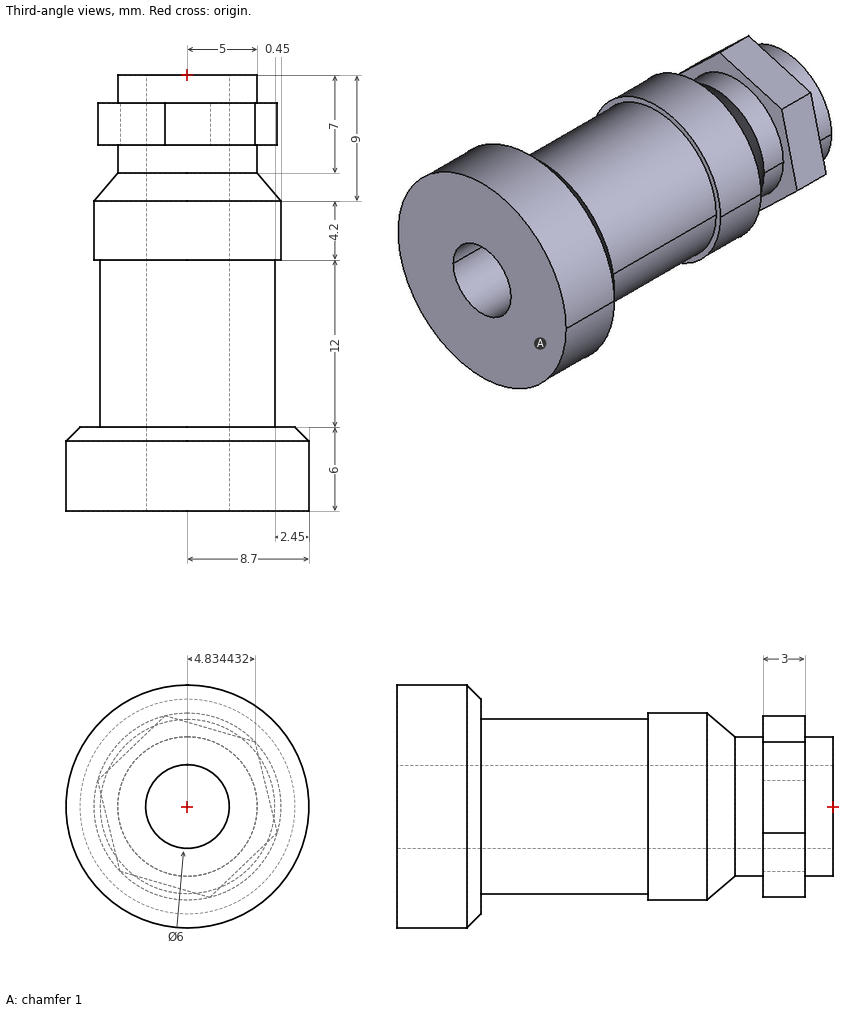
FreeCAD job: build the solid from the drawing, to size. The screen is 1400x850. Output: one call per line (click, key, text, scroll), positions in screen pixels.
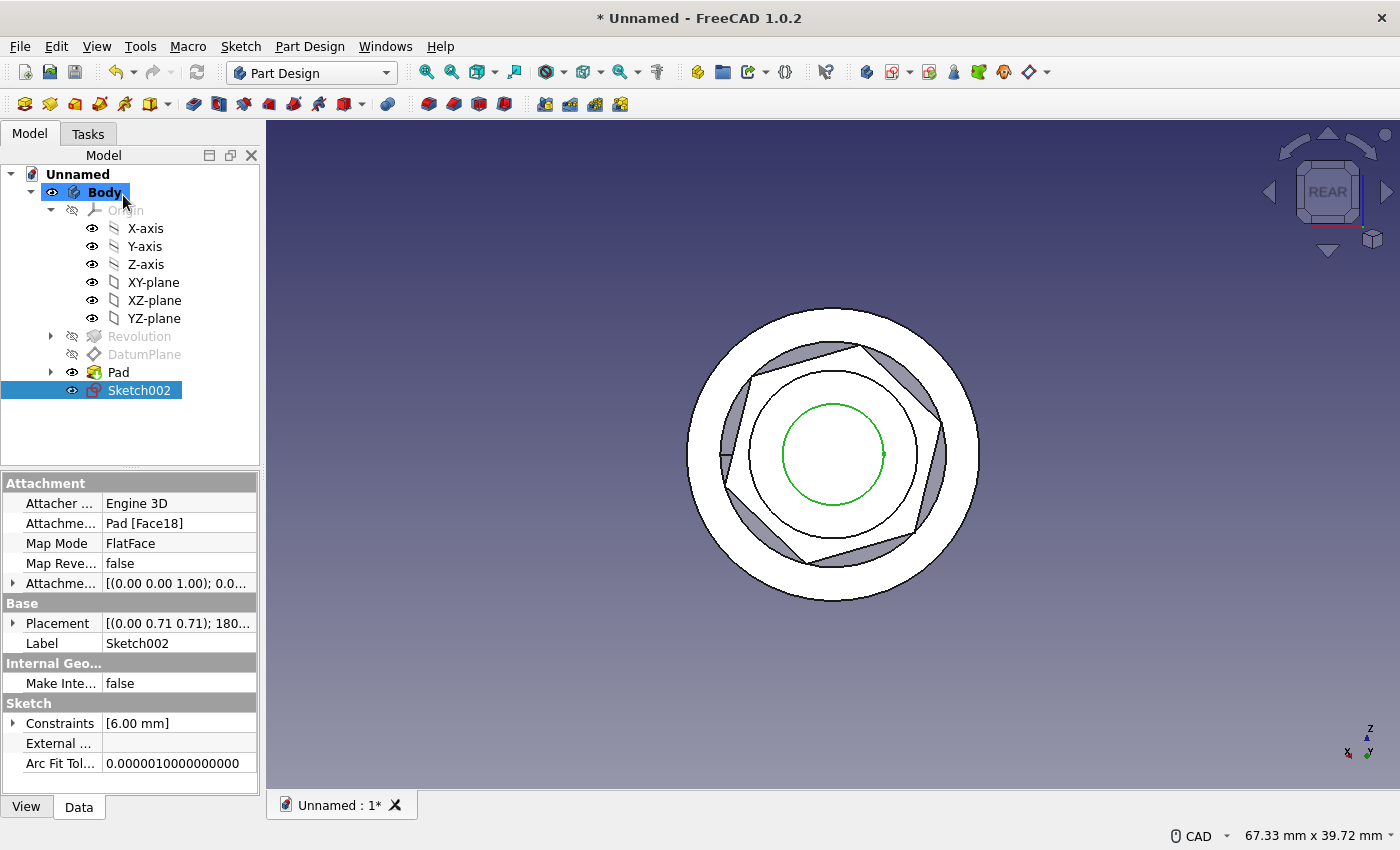
click(194, 104)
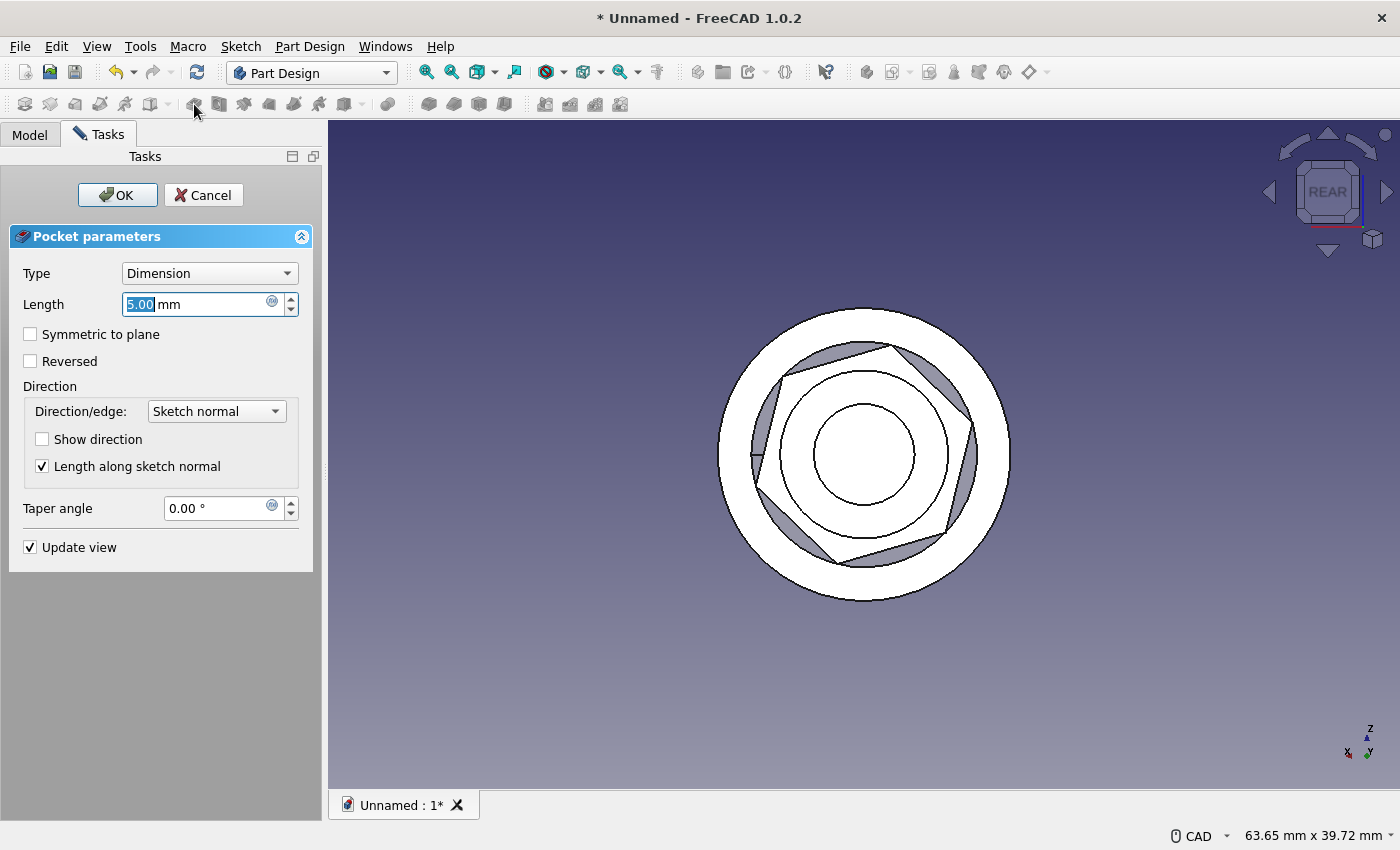
click(210, 274)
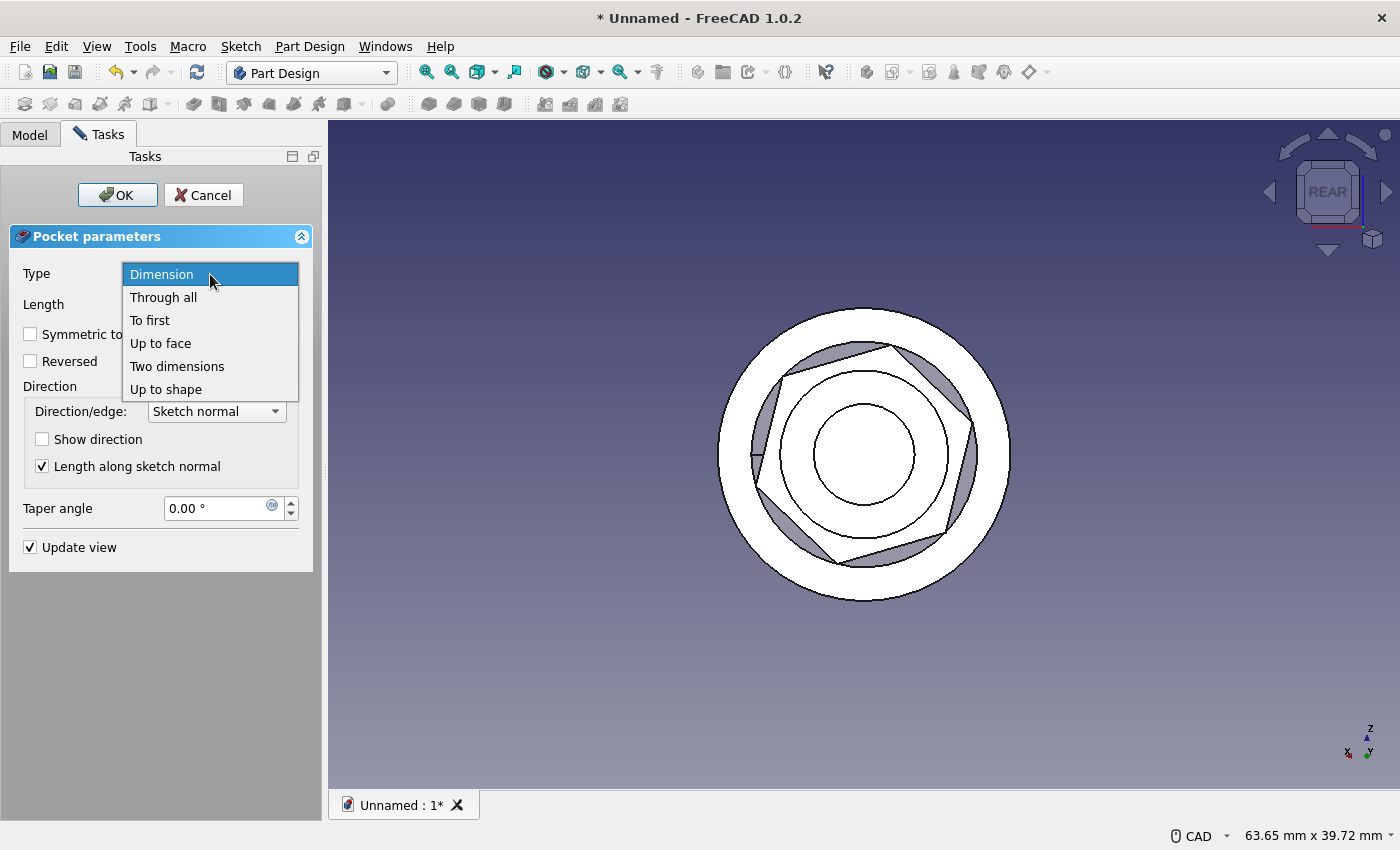
click(208, 298)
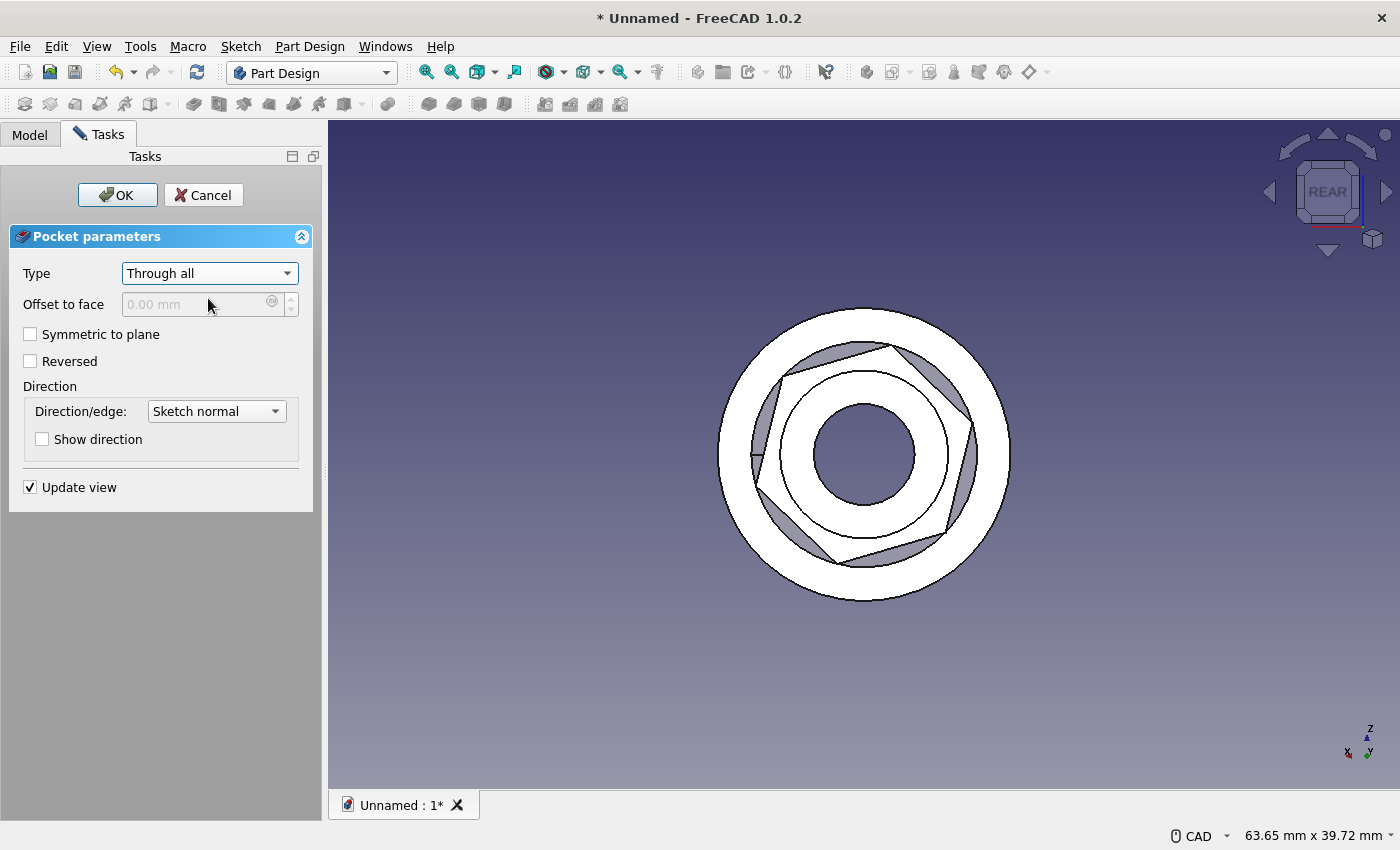
click(118, 195)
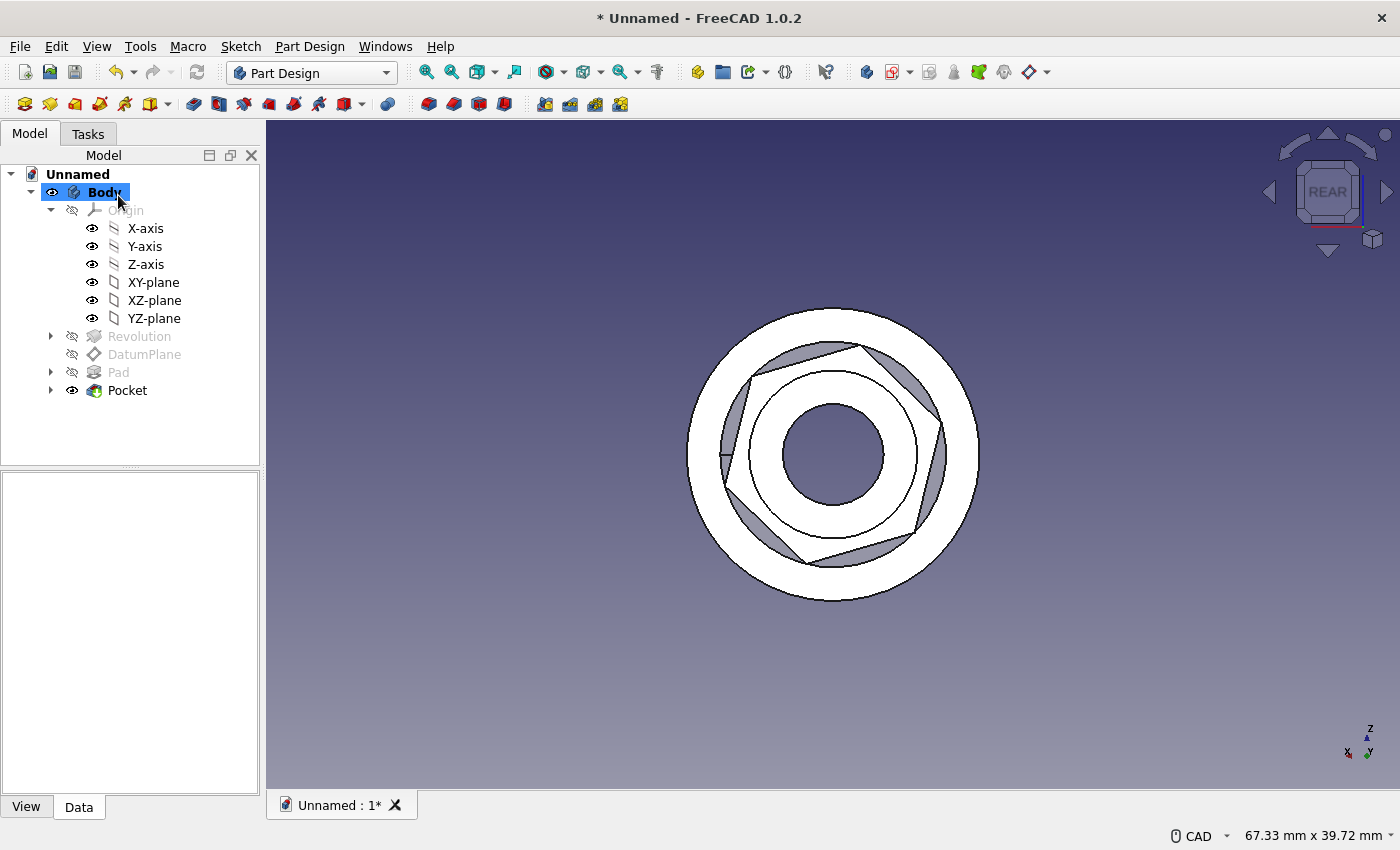
key(v)
key(f)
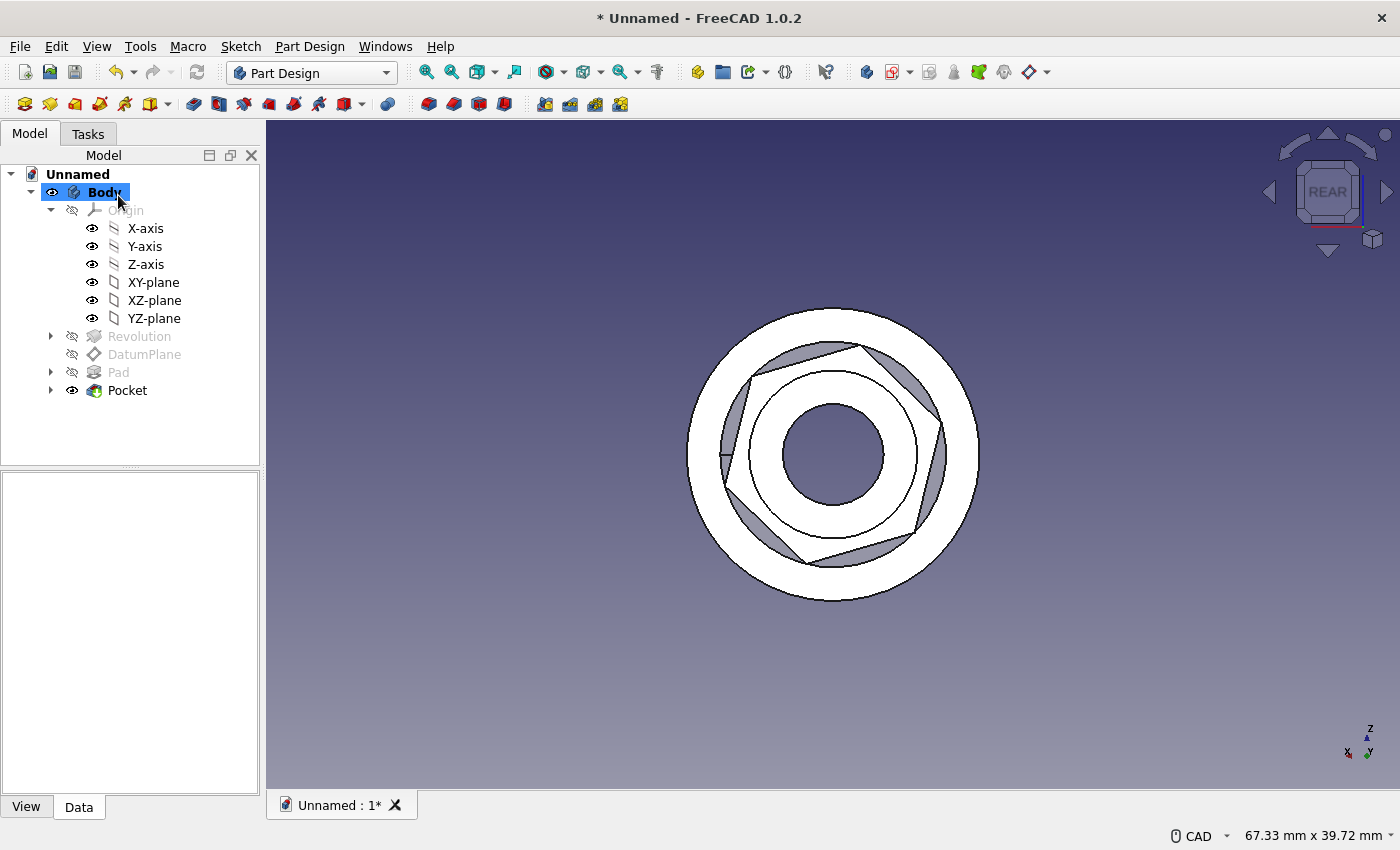
click(980, 453)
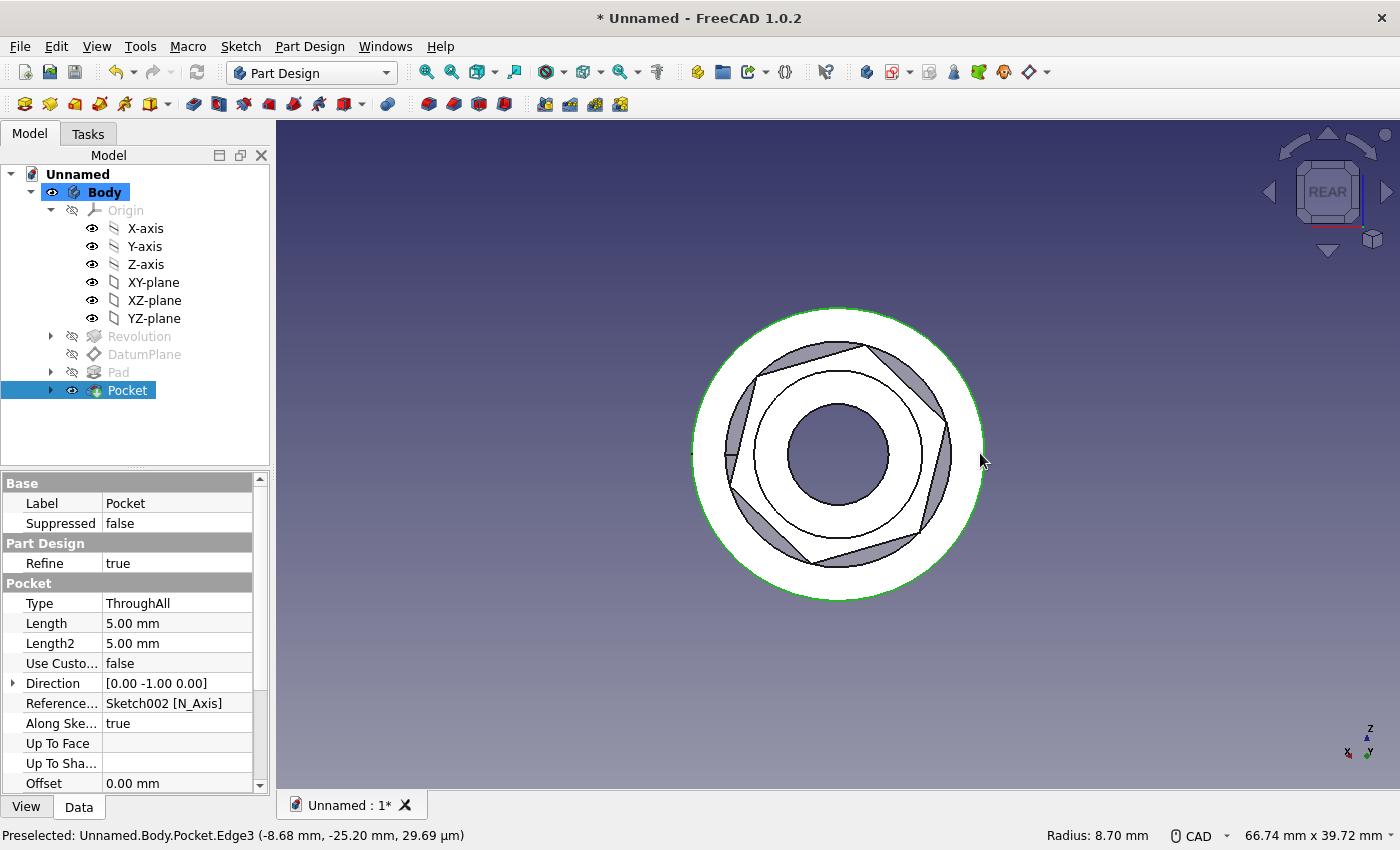
click(454, 104)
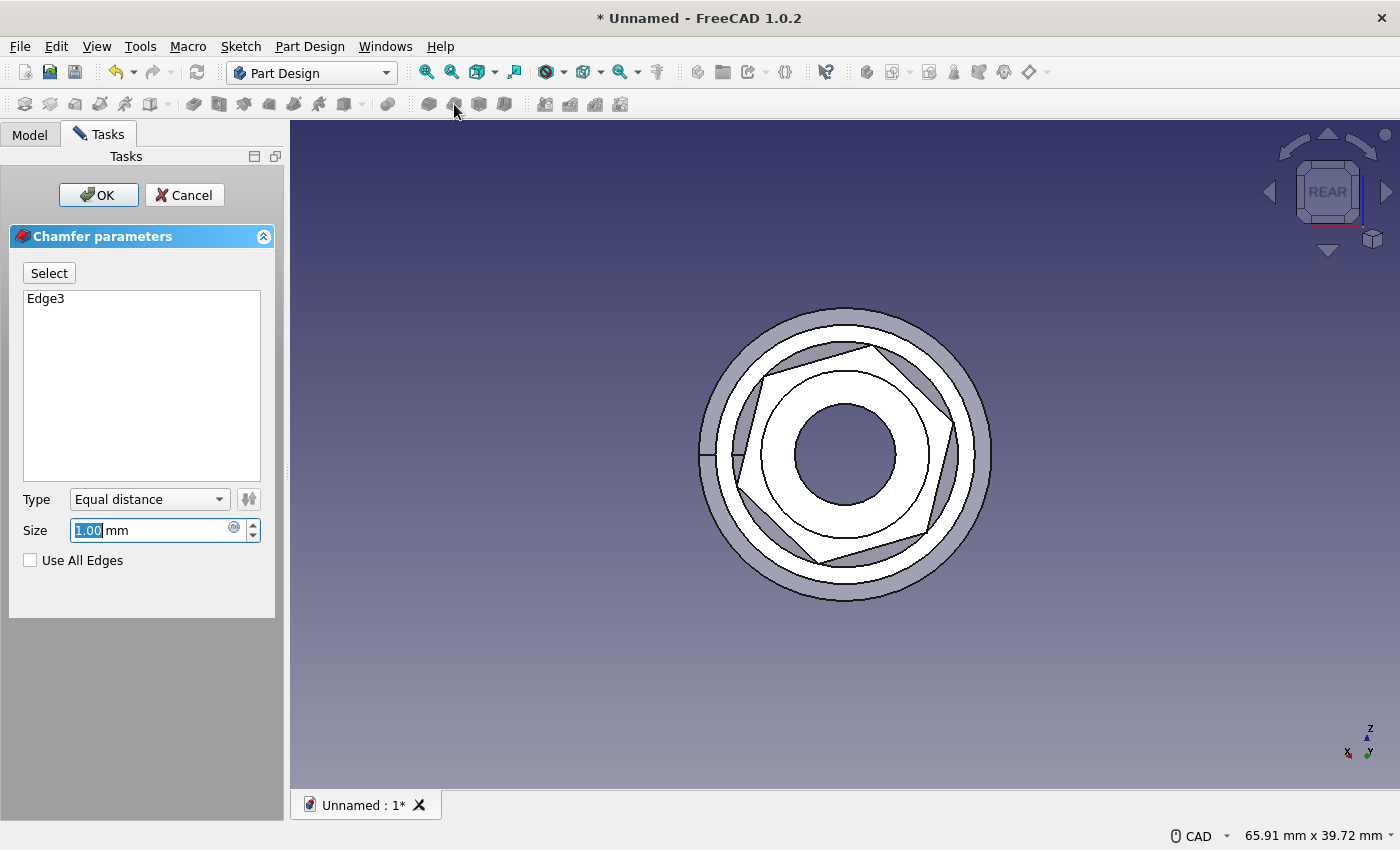
text(1)
key(Tab)